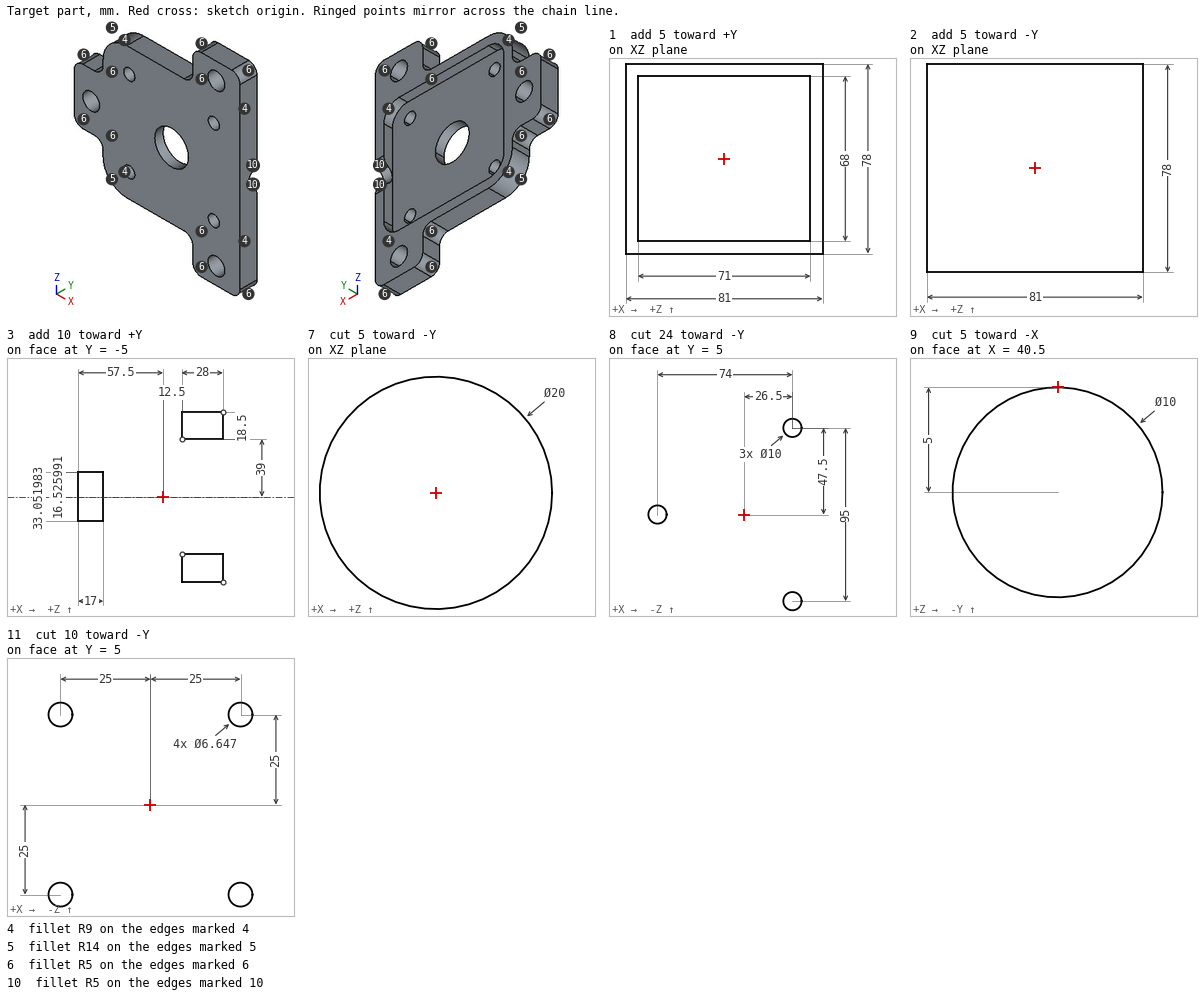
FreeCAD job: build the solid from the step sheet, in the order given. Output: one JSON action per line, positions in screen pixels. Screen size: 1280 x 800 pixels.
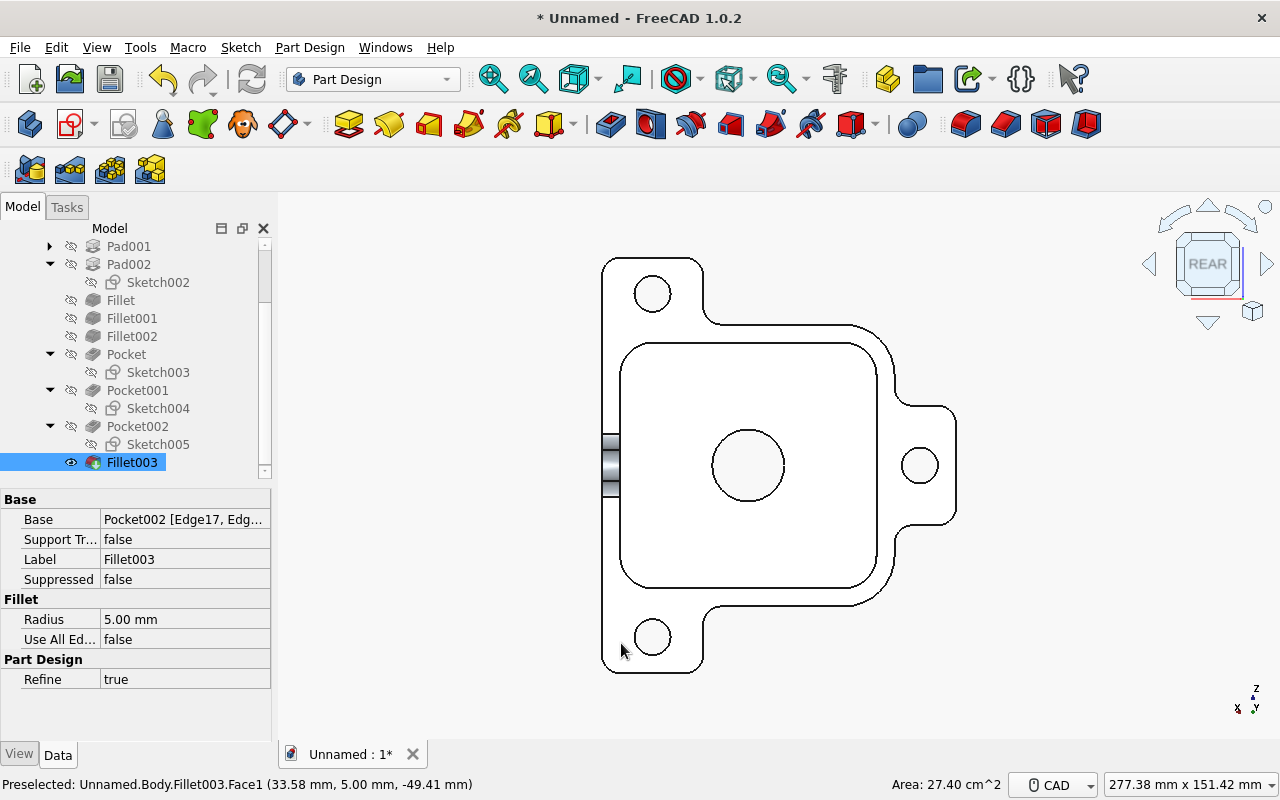
{"action": "left_click", "coordinate": [70, 124]}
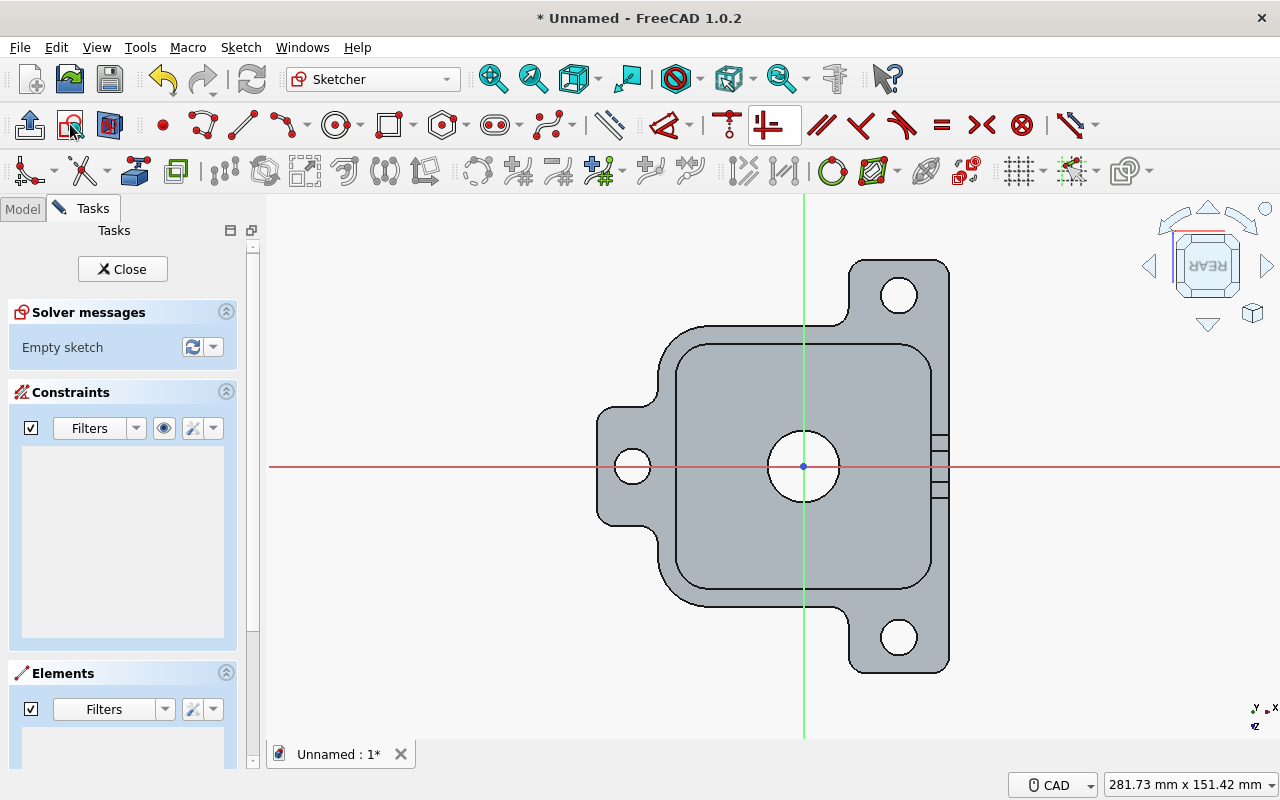
{"action": "scroll", "coordinate": [924, 467], "scroll_direction": "up", "scroll_amount": 3}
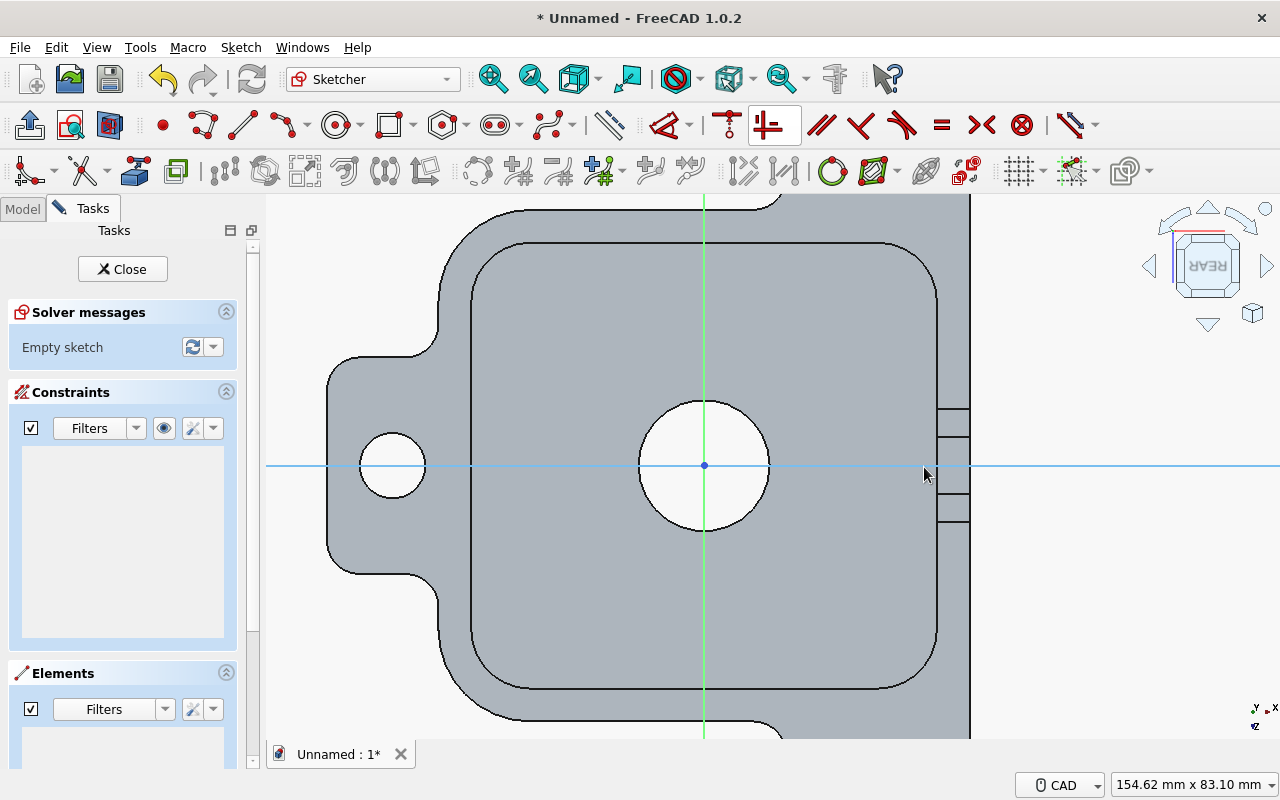
{"action": "left_click", "coordinate": [336, 126]}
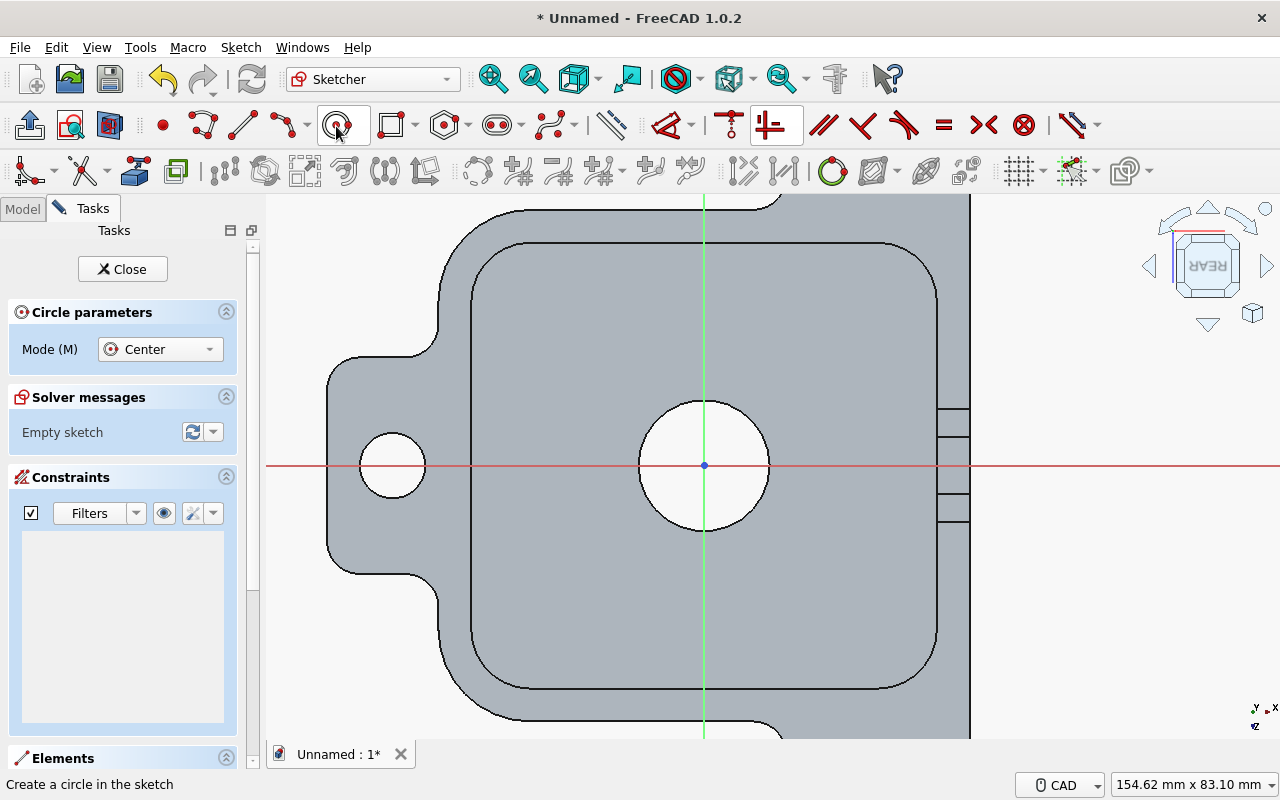
{"action": "left_click", "coordinate": [868, 302]}
{"action": "left_click", "coordinate": [883, 286]}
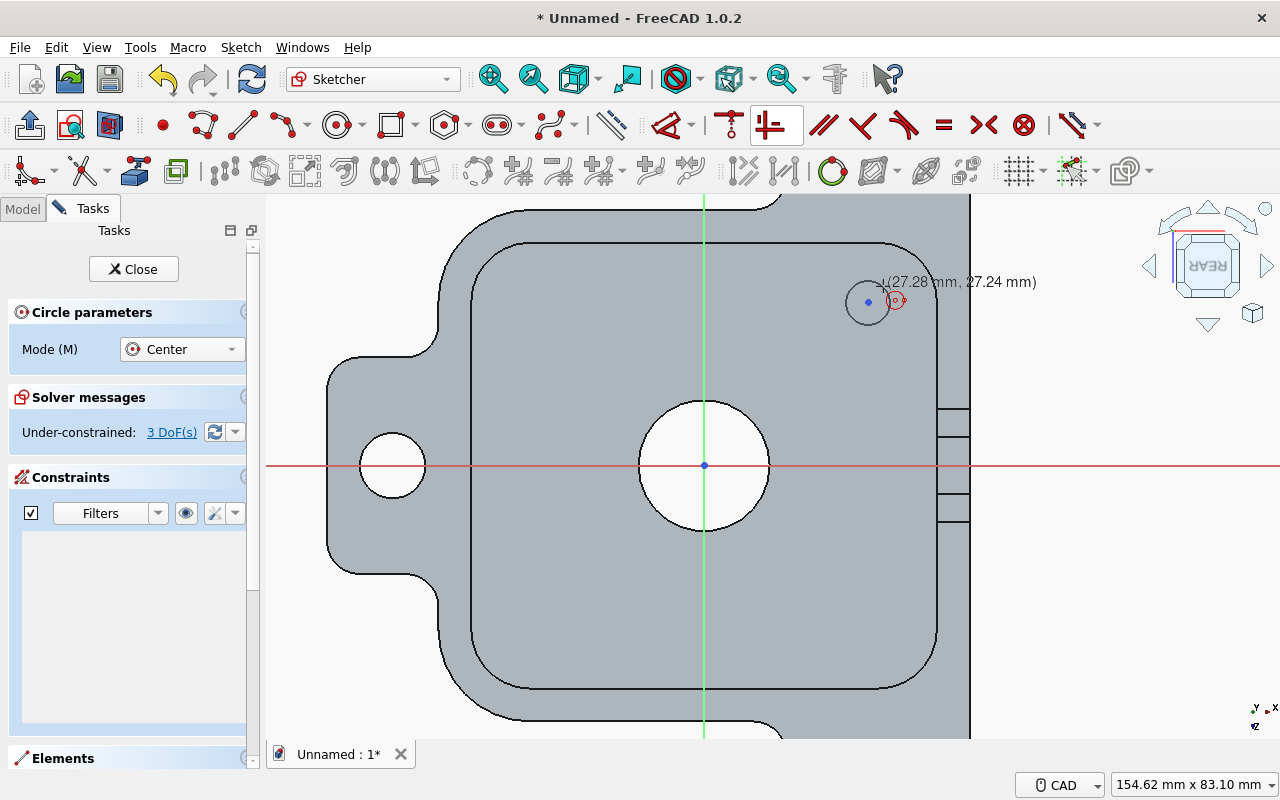
{"action": "left_click", "coordinate": [540, 302]}
{"action": "left_click", "coordinate": [556, 286]}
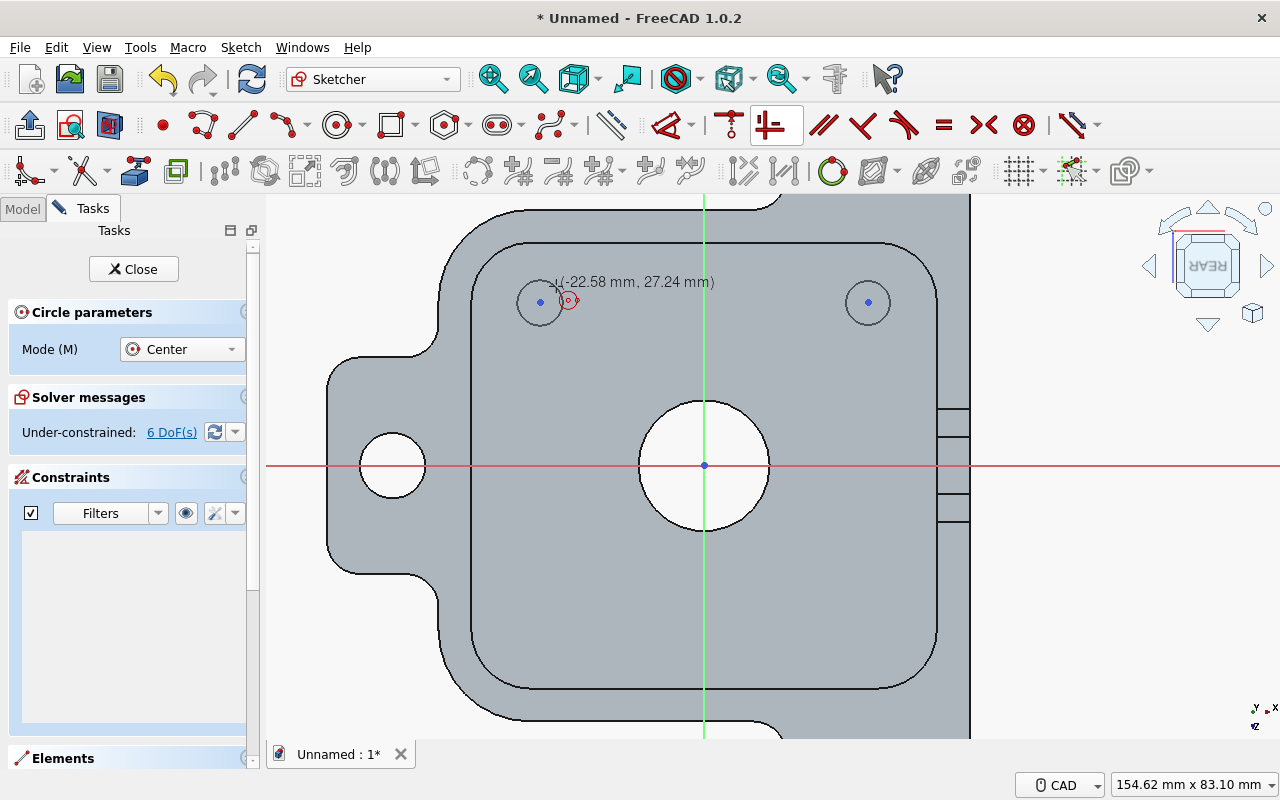
{"action": "left_click", "coordinate": [540, 630]}
{"action": "left_click", "coordinate": [556, 614]}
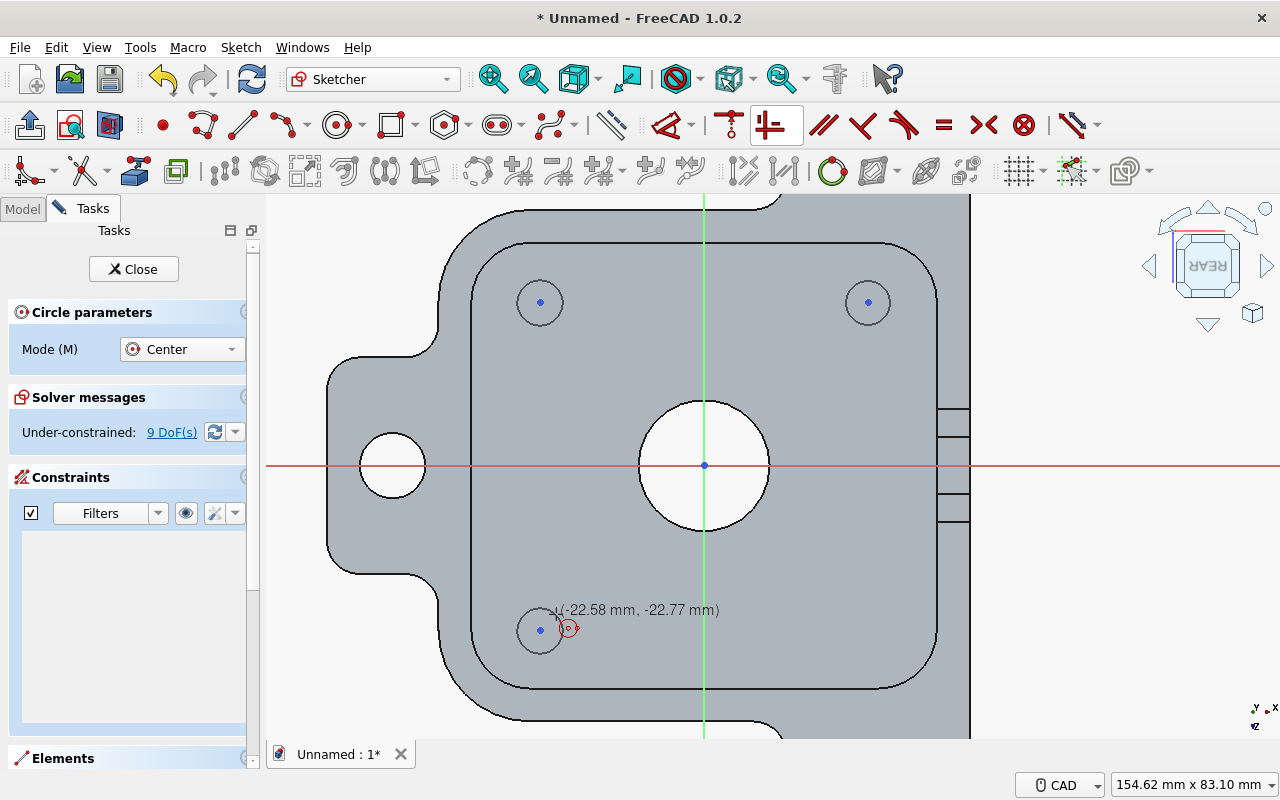
{"action": "left_click", "coordinate": [868, 630]}
{"action": "left_click", "coordinate": [883, 614]}
{"action": "key", "text": "Escape"}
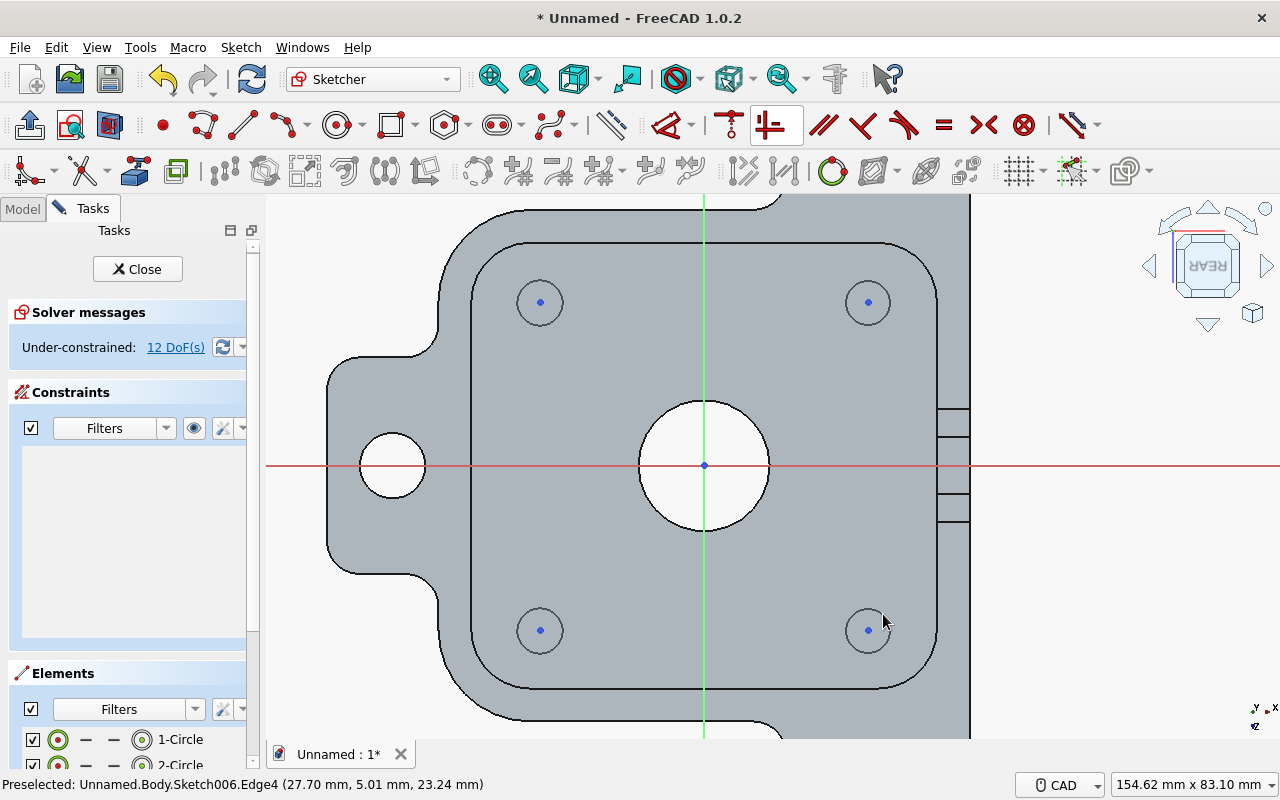
{"action": "left_click", "coordinate": [883, 287]}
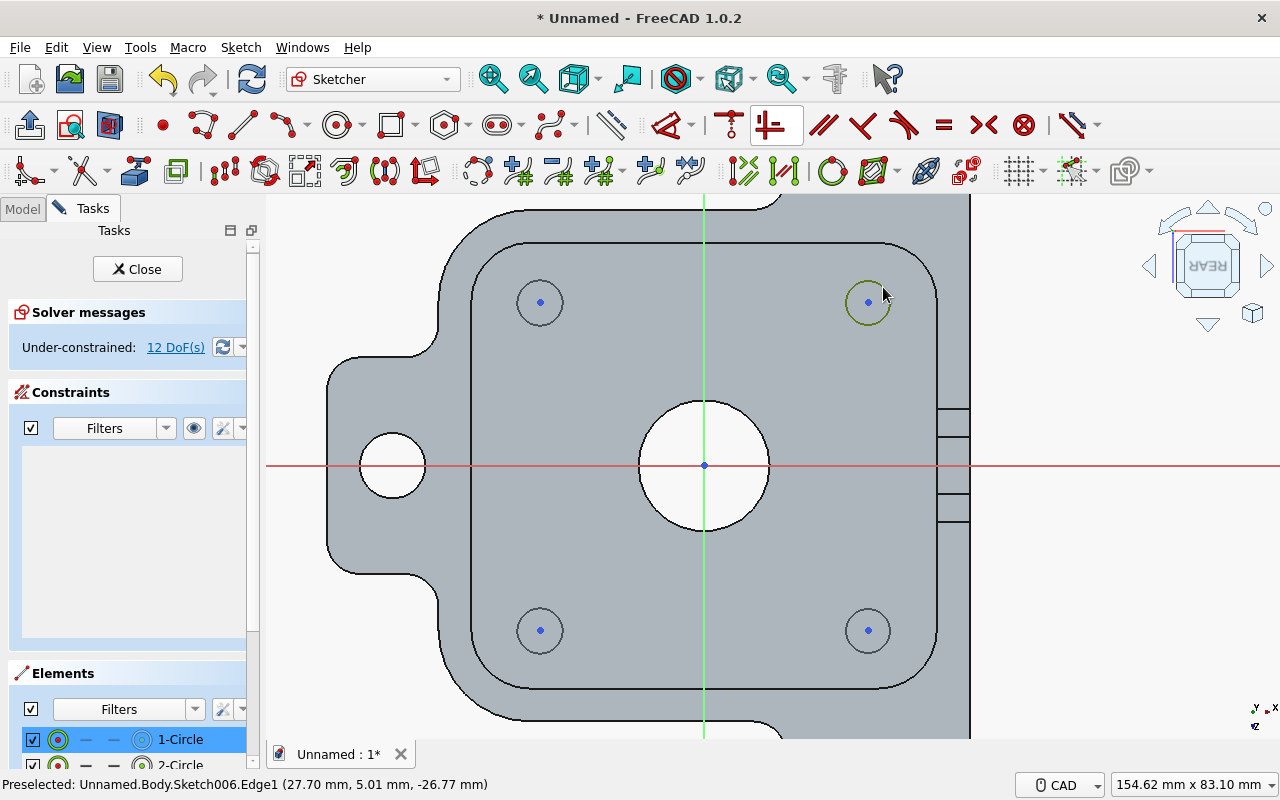
{"action": "left_click", "coordinate": [556, 287]}